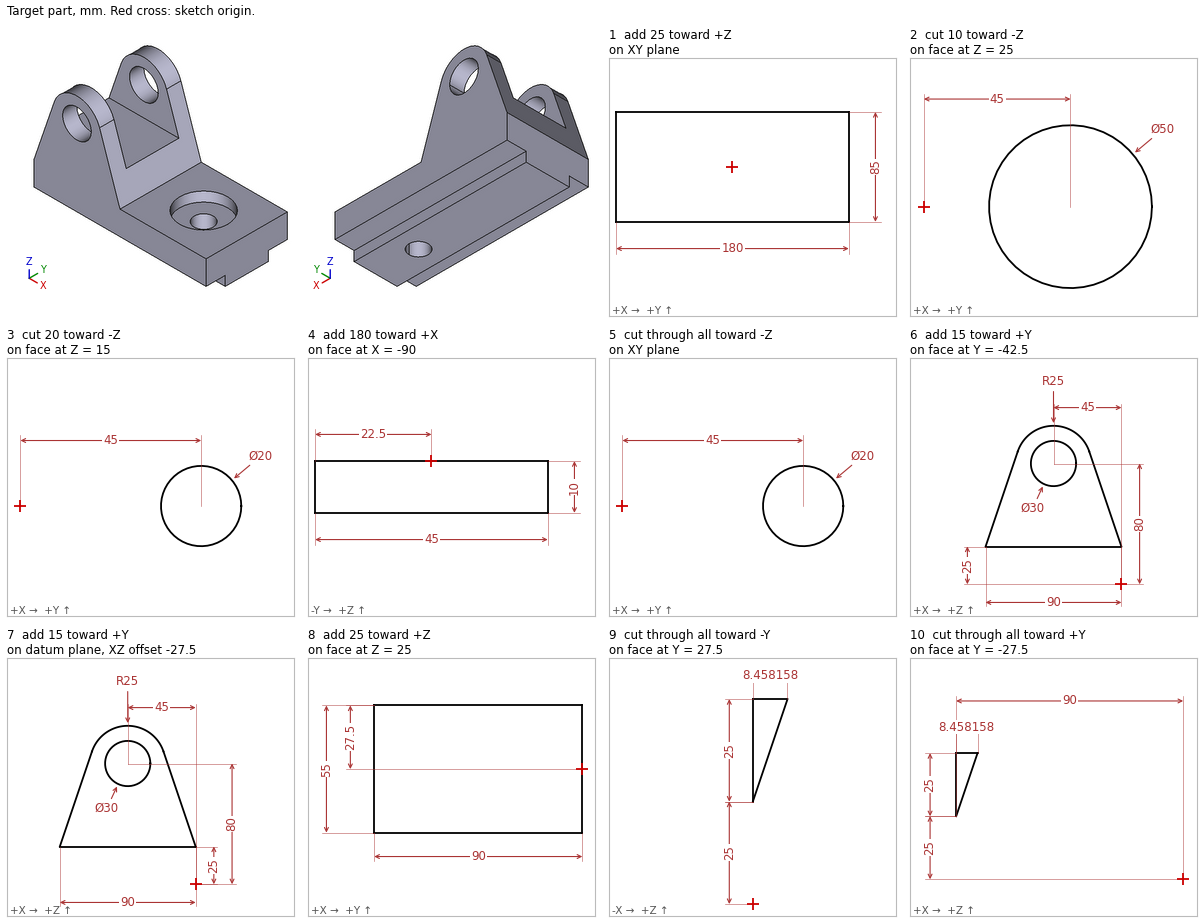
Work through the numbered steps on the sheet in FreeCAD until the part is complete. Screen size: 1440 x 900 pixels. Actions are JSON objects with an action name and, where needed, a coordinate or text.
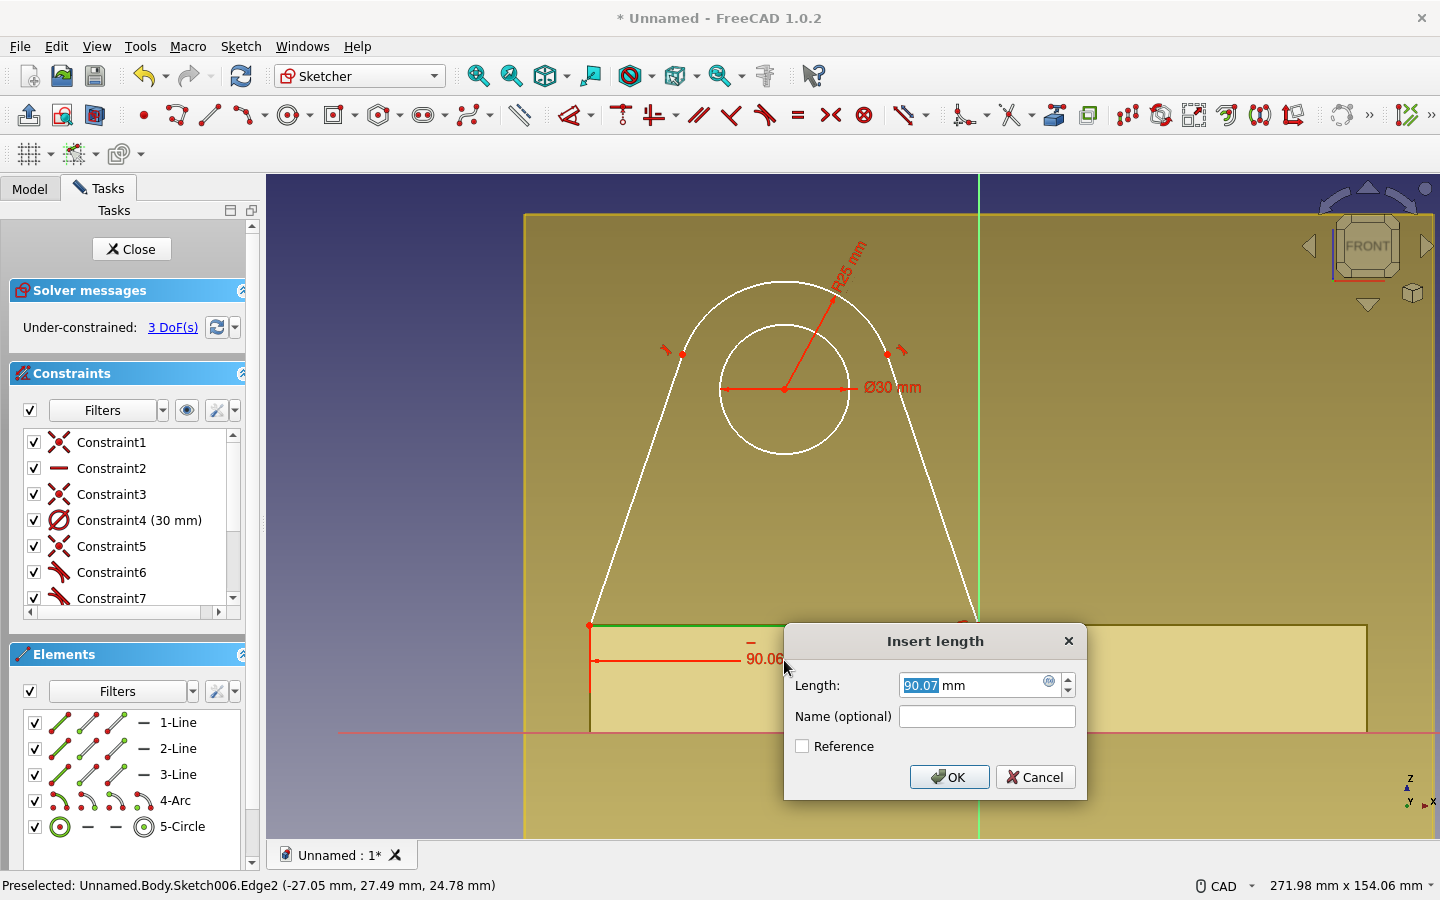
{"action": "type", "text": "90"}
{"action": "key", "text": "Return"}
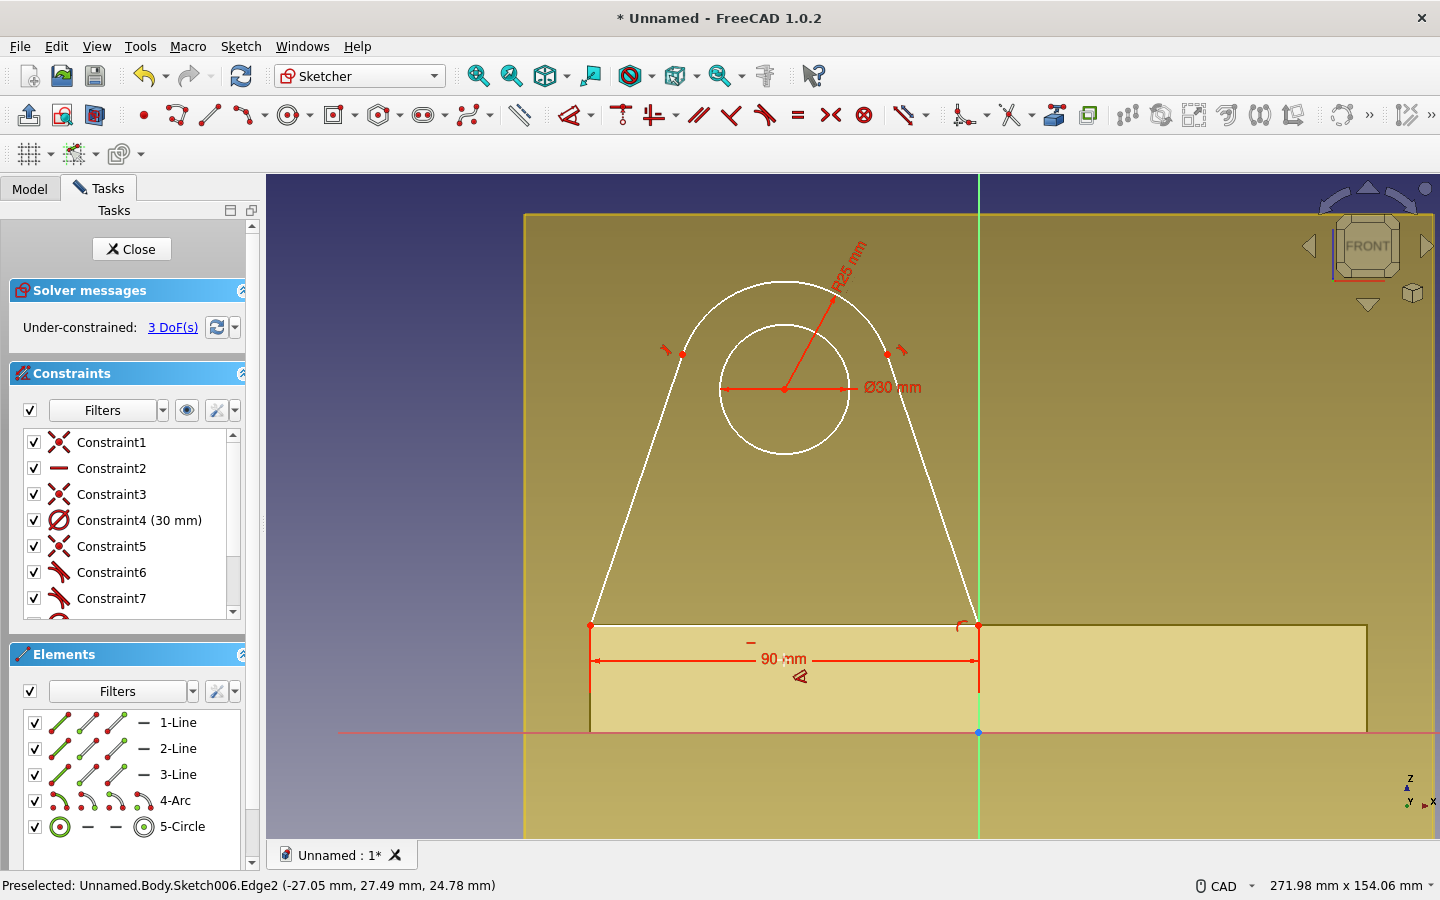
{"action": "left_click", "coordinate": [785, 389]}
{"action": "left_click", "coordinate": [882, 767]}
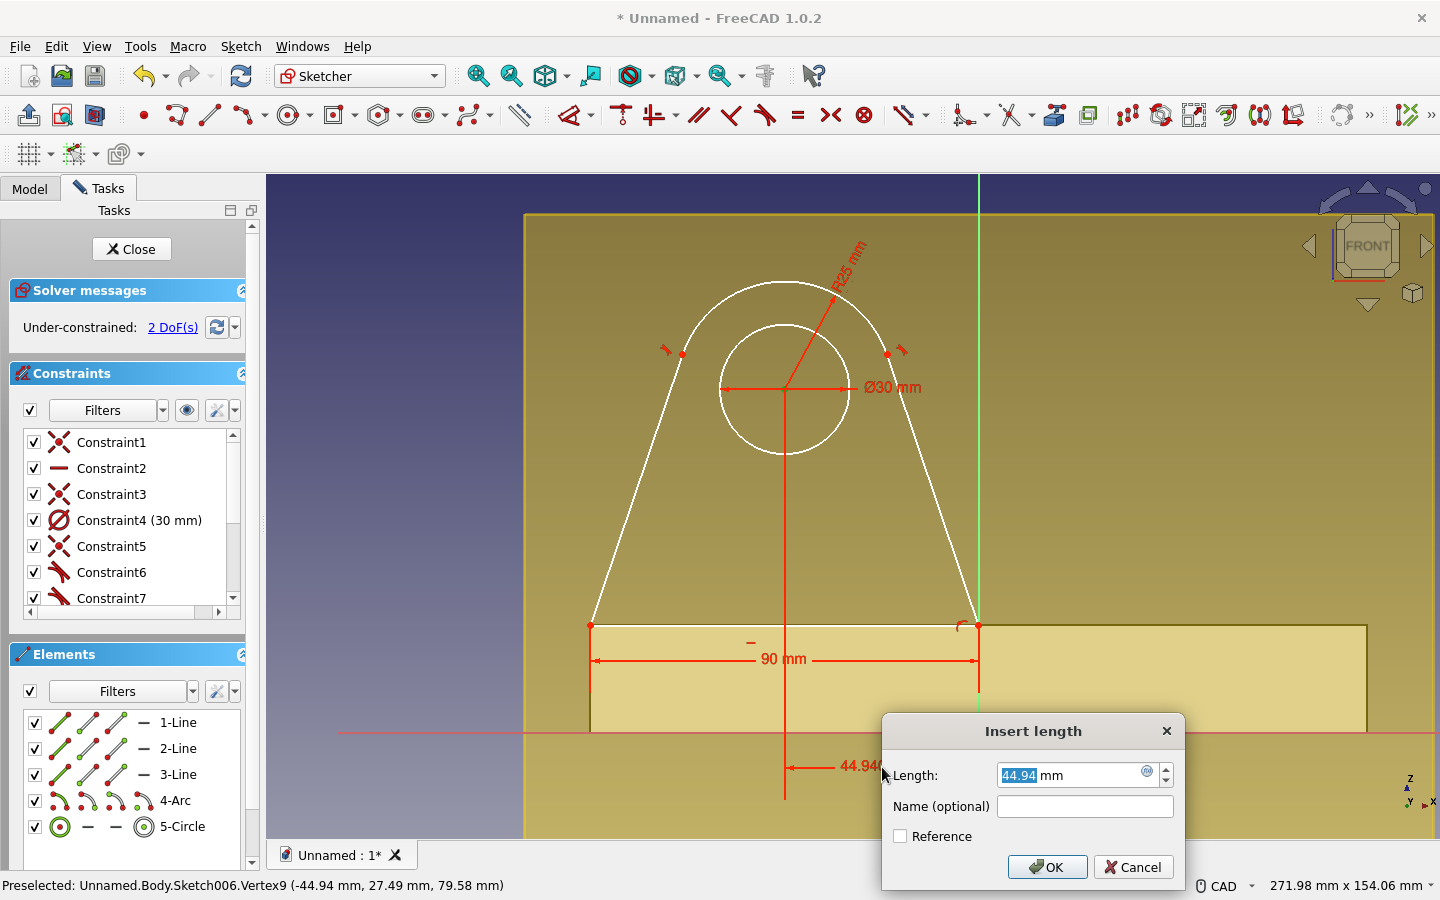
{"action": "type", "text": "45"}
{"action": "key", "text": "Return"}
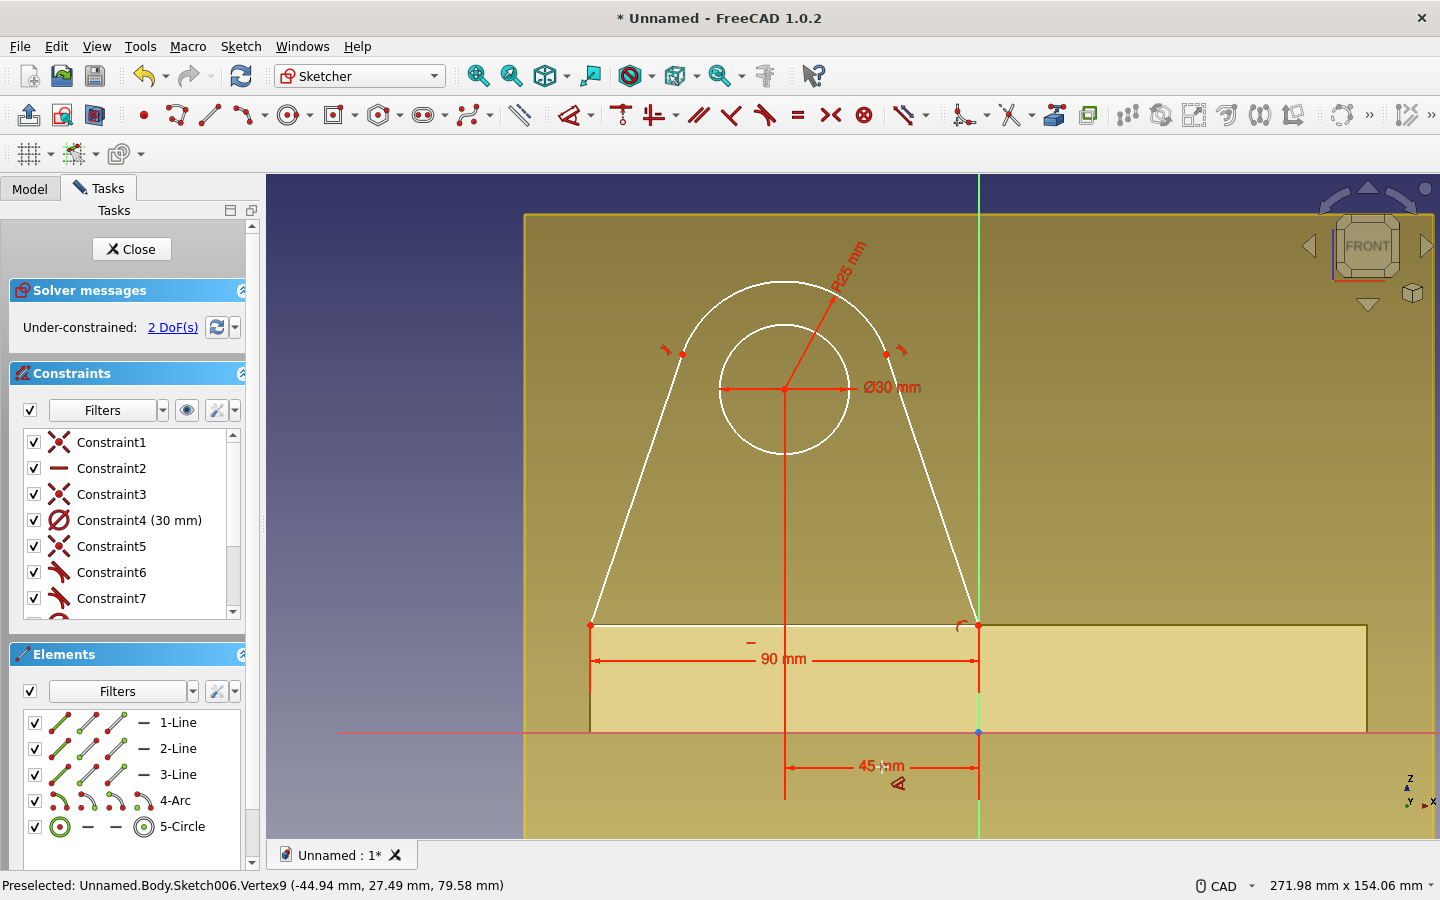
{"action": "left_click", "coordinate": [785, 389]}
{"action": "left_click", "coordinate": [1013, 561]}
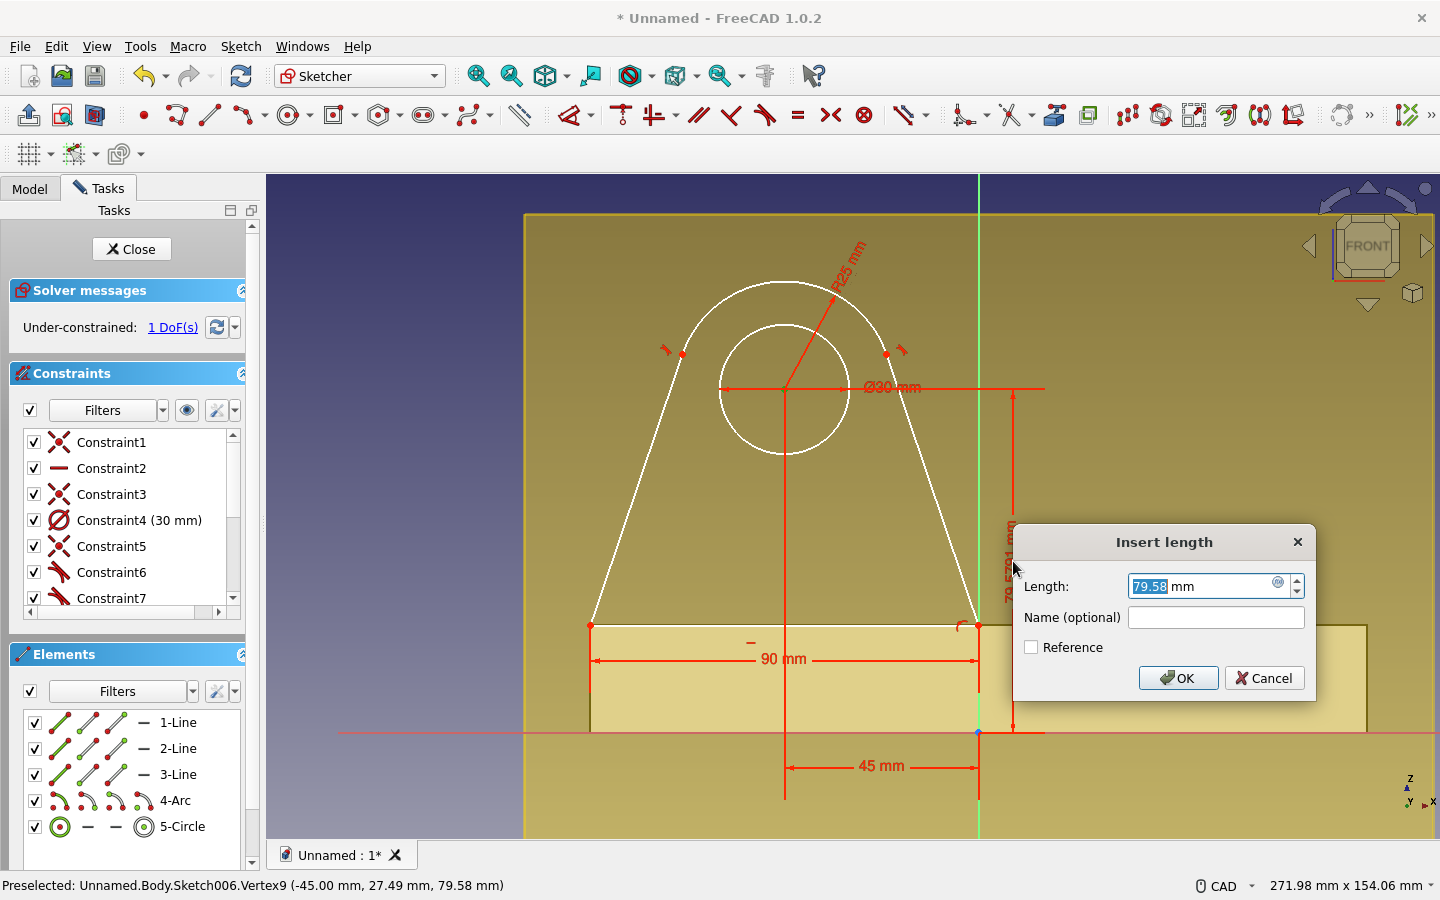
{"action": "type", "text": "80"}
{"action": "key", "text": "Return"}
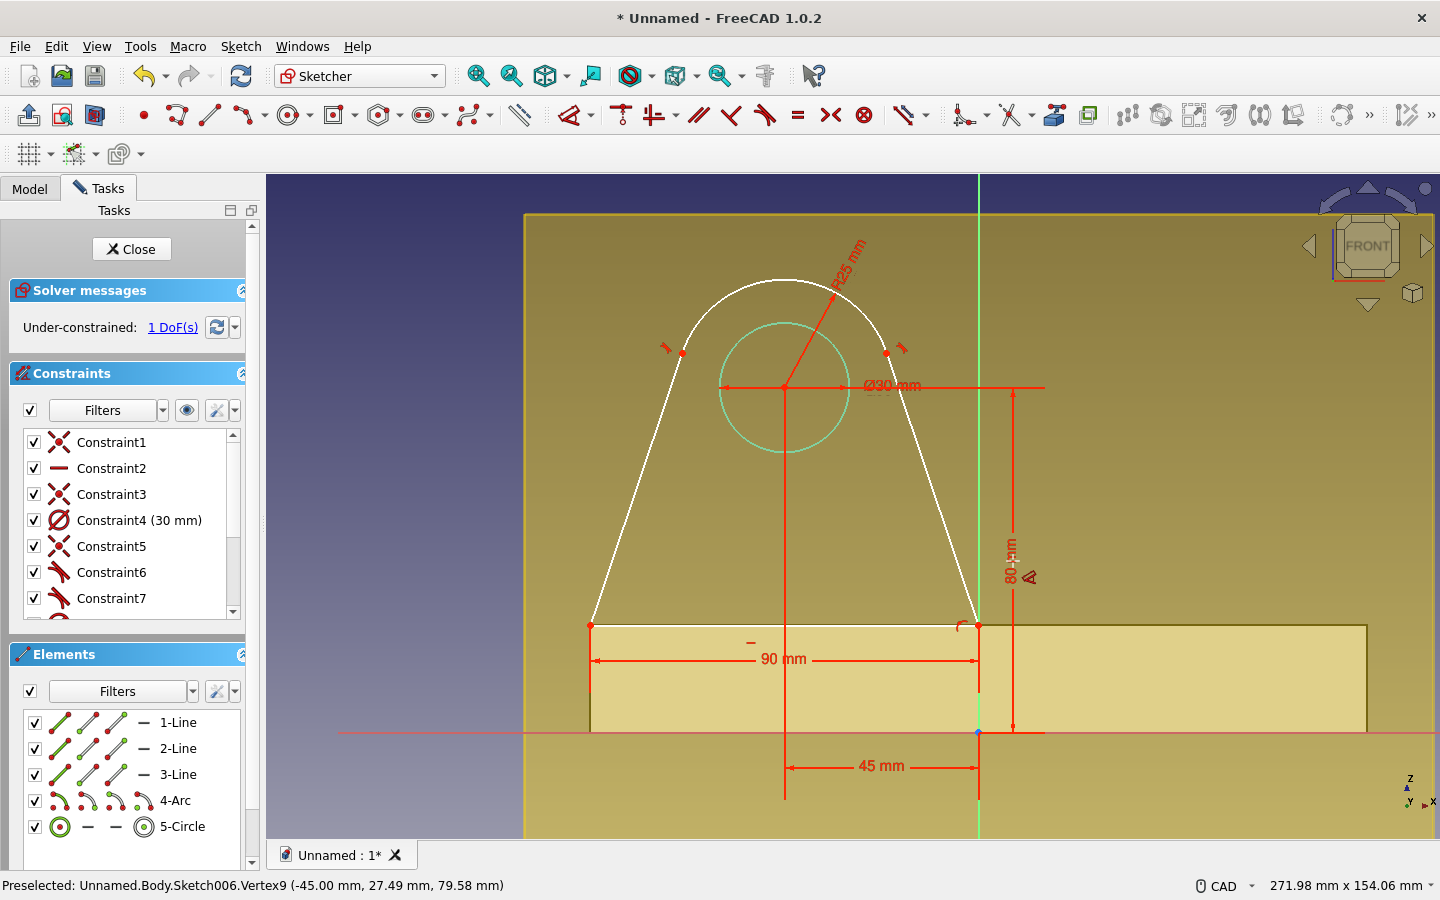
{"action": "left_click", "coordinate": [979, 626]}
{"action": "left_click", "coordinate": [1013, 679]}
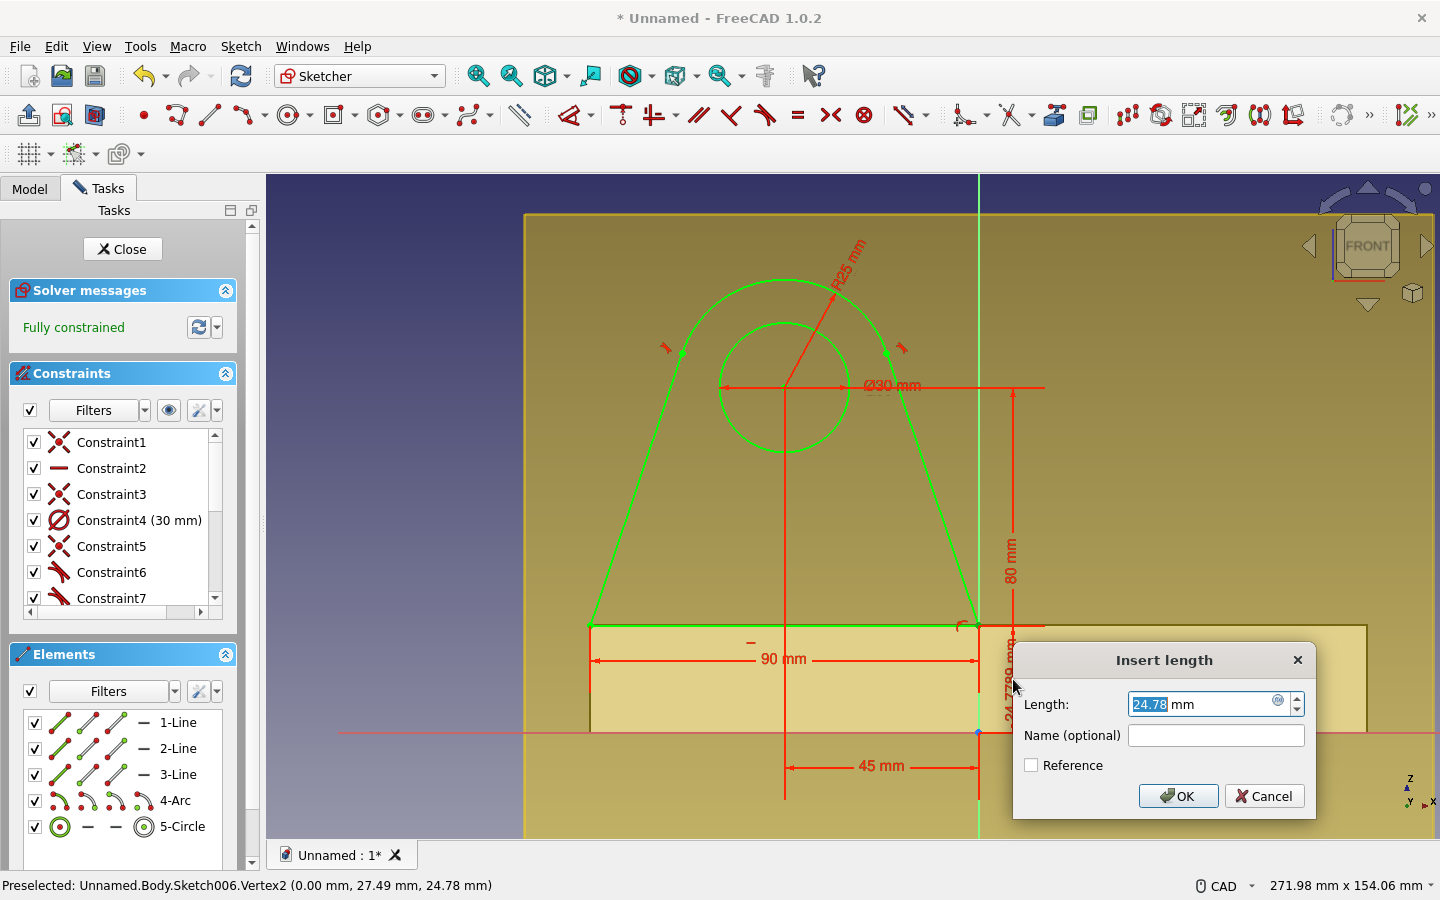
{"action": "type", "text": "25"}
{"action": "key", "text": "Return"}
{"action": "key", "text": "Escape"}